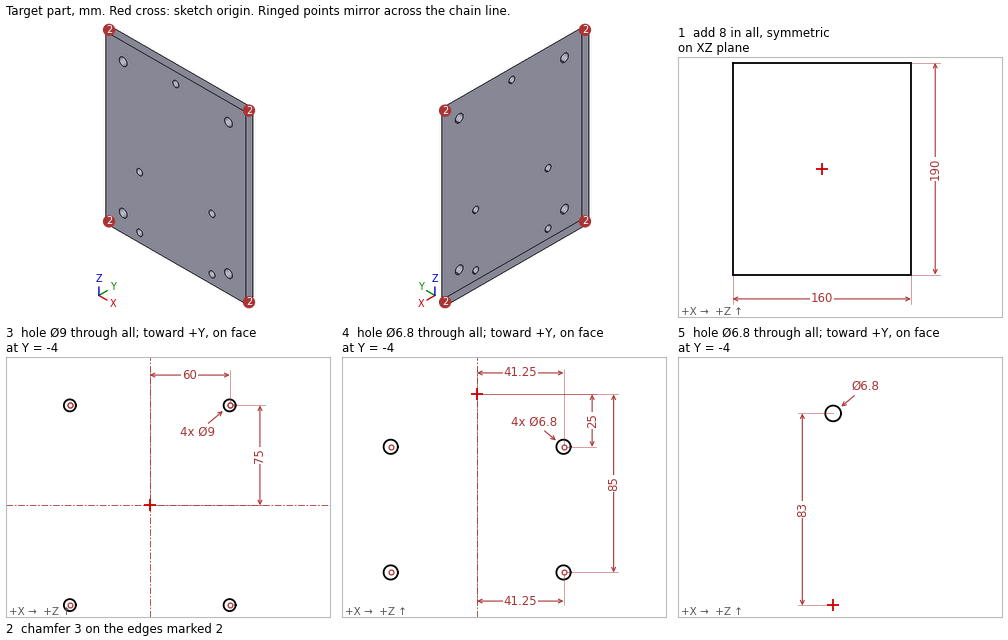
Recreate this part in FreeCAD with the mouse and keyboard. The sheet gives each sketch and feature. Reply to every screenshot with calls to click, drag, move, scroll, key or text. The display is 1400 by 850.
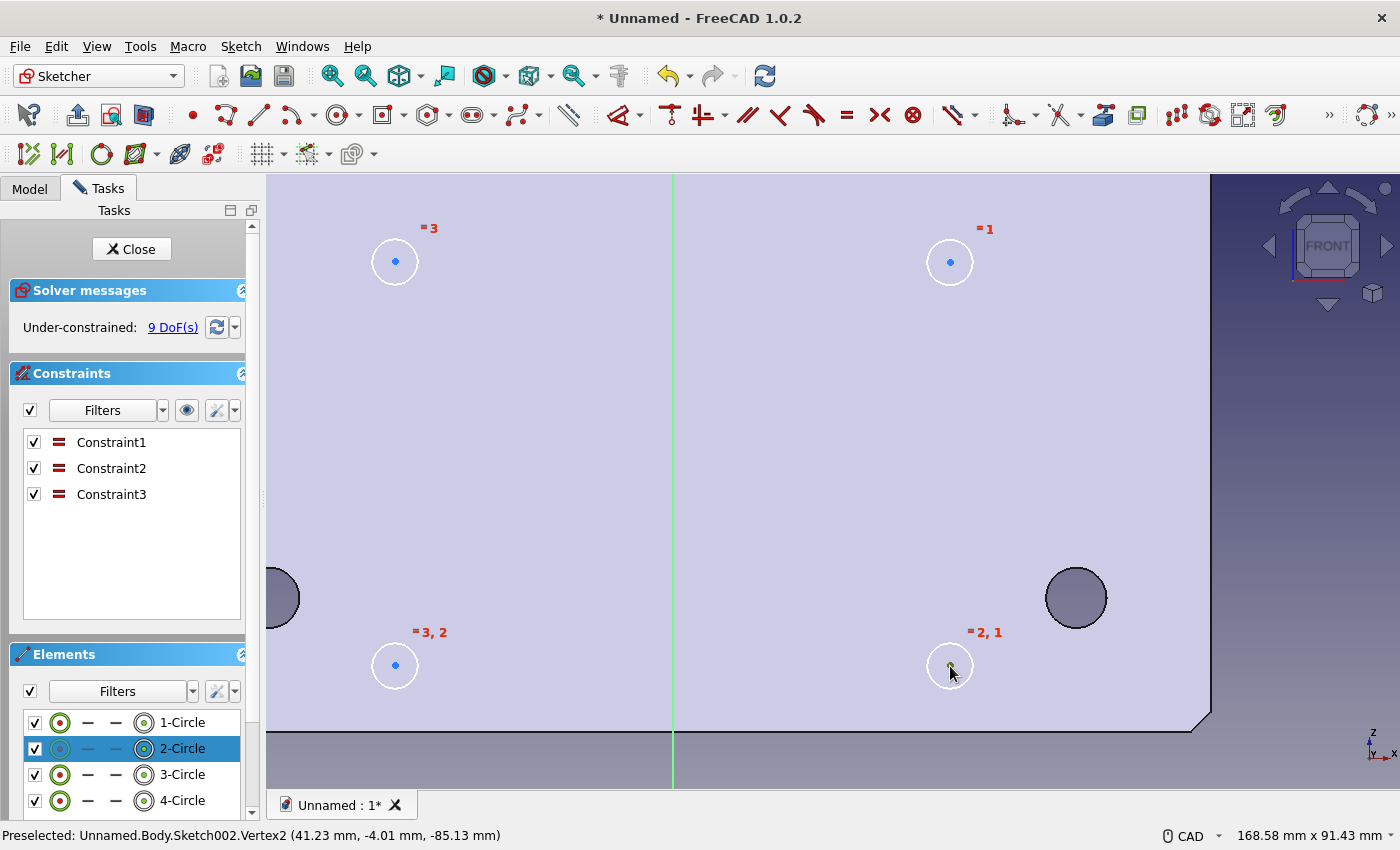
click(395, 666)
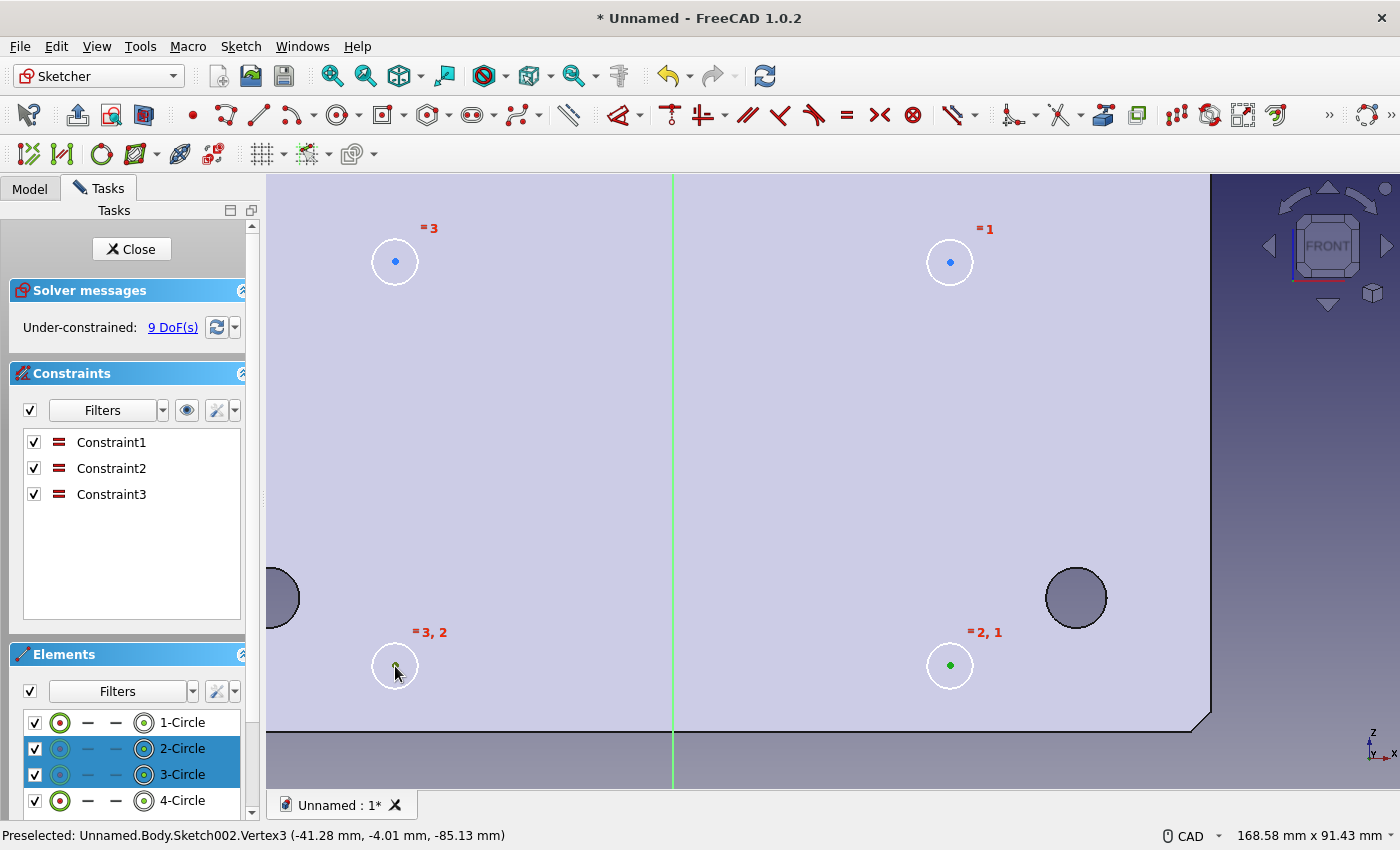
click(673, 721)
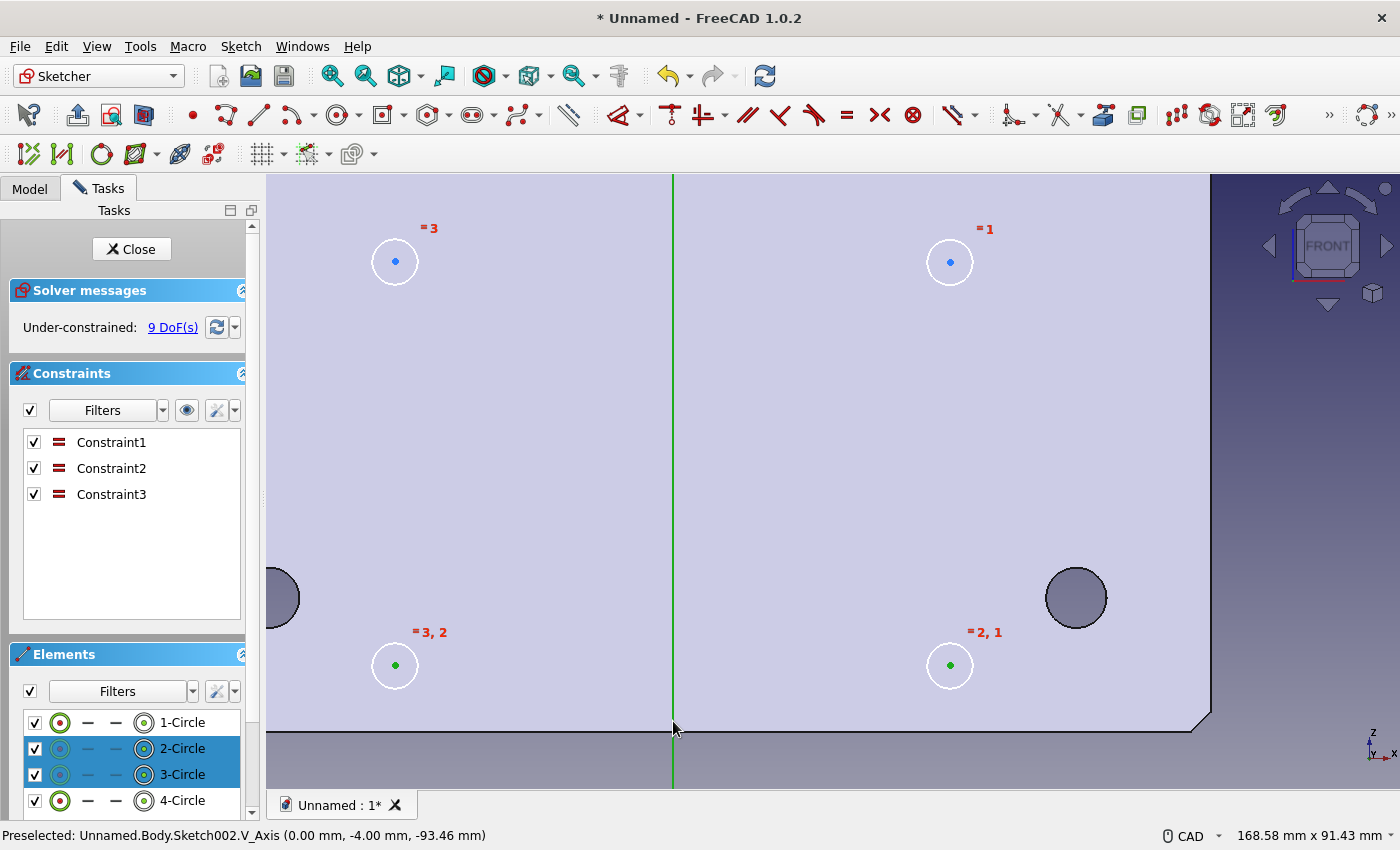
click(880, 116)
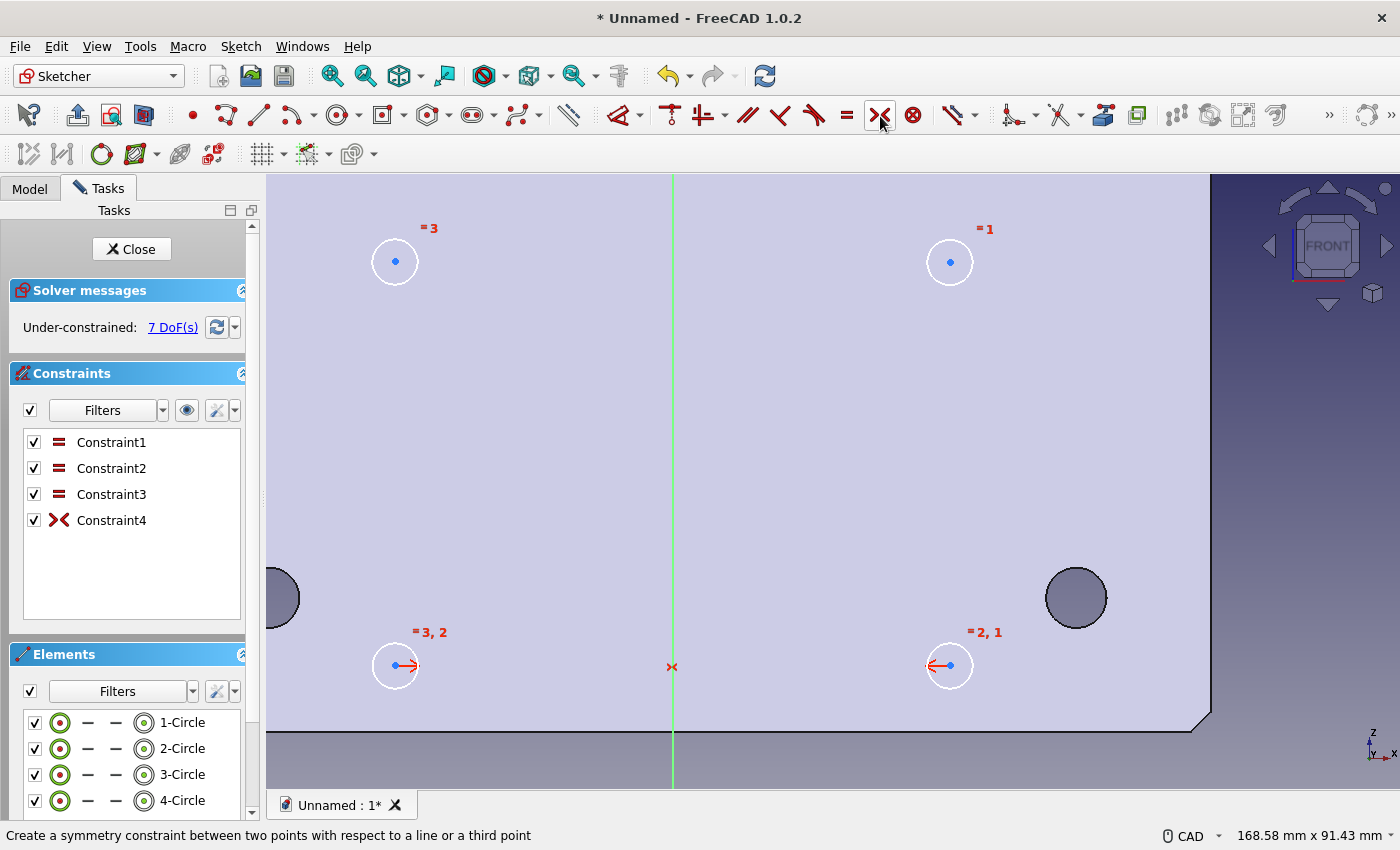
click(950, 262)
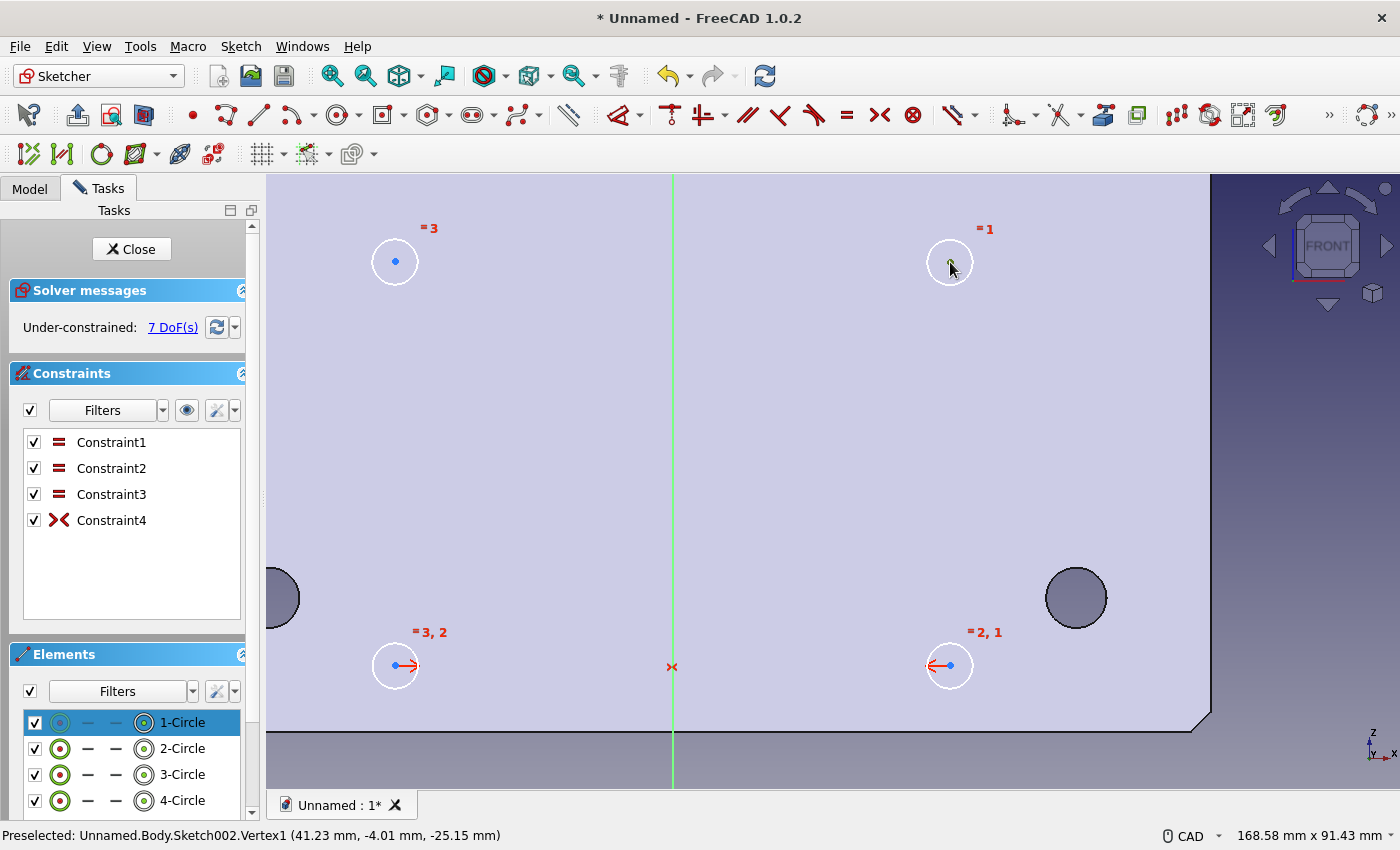
click(395, 262)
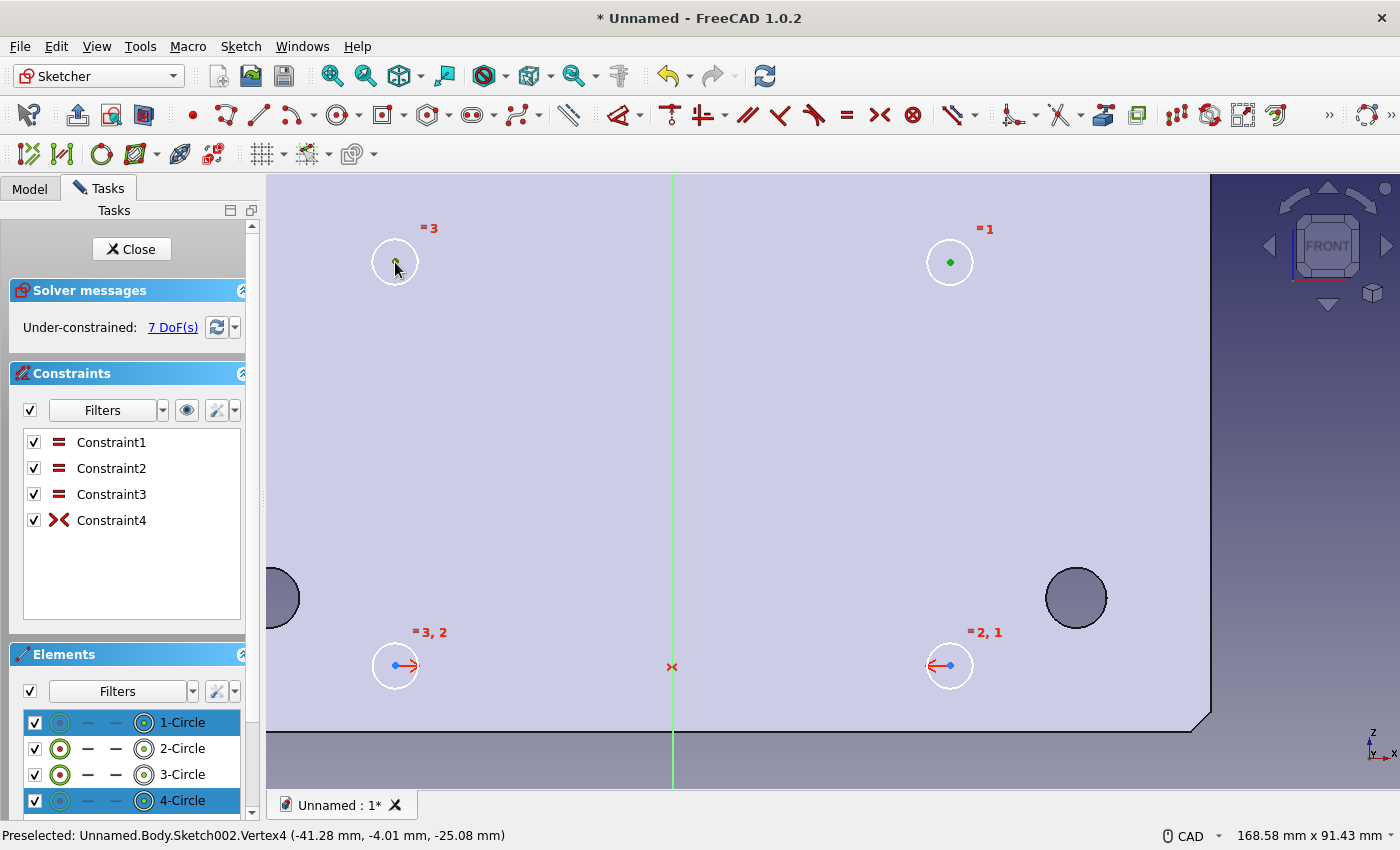
click(673, 721)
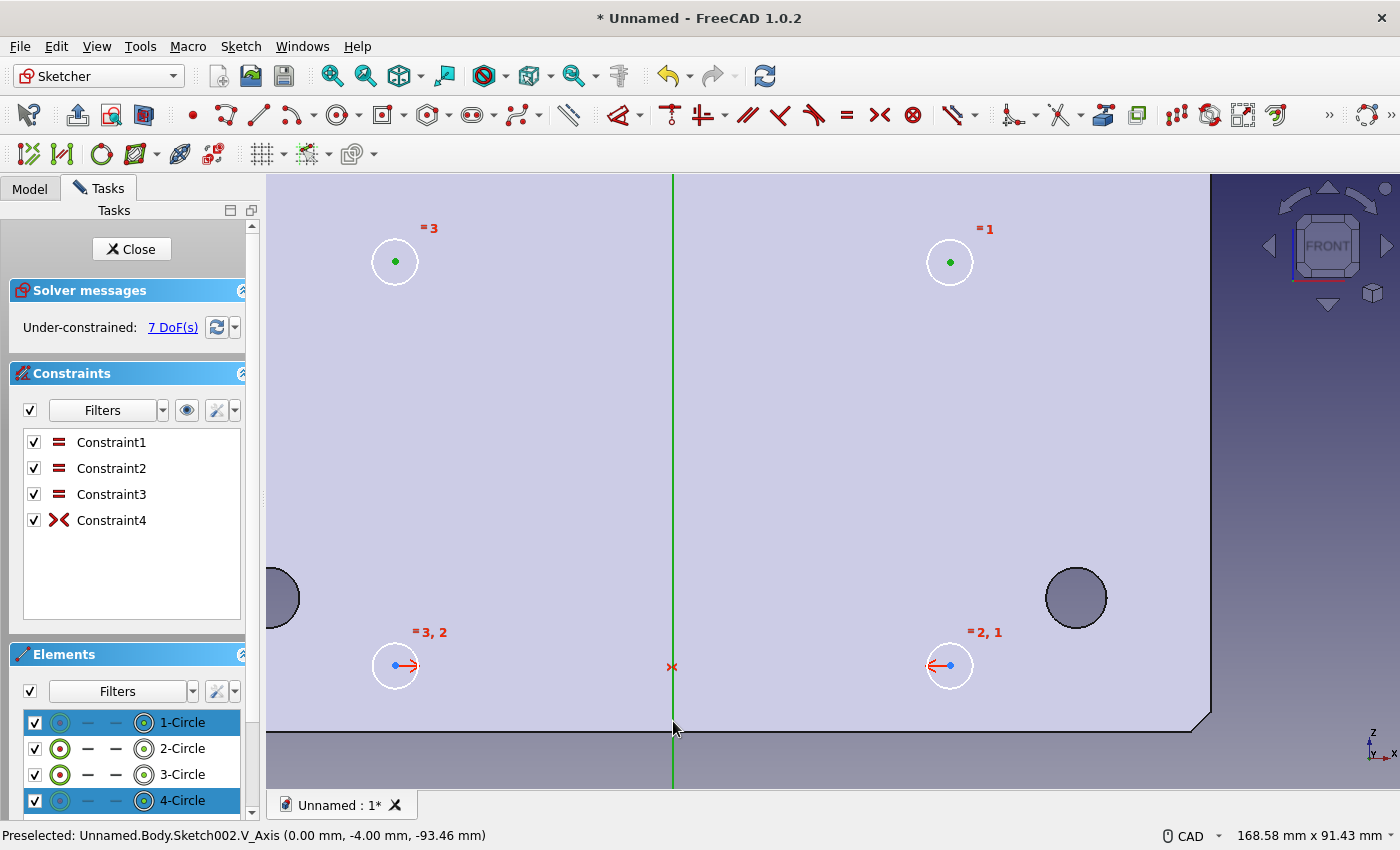
click(880, 116)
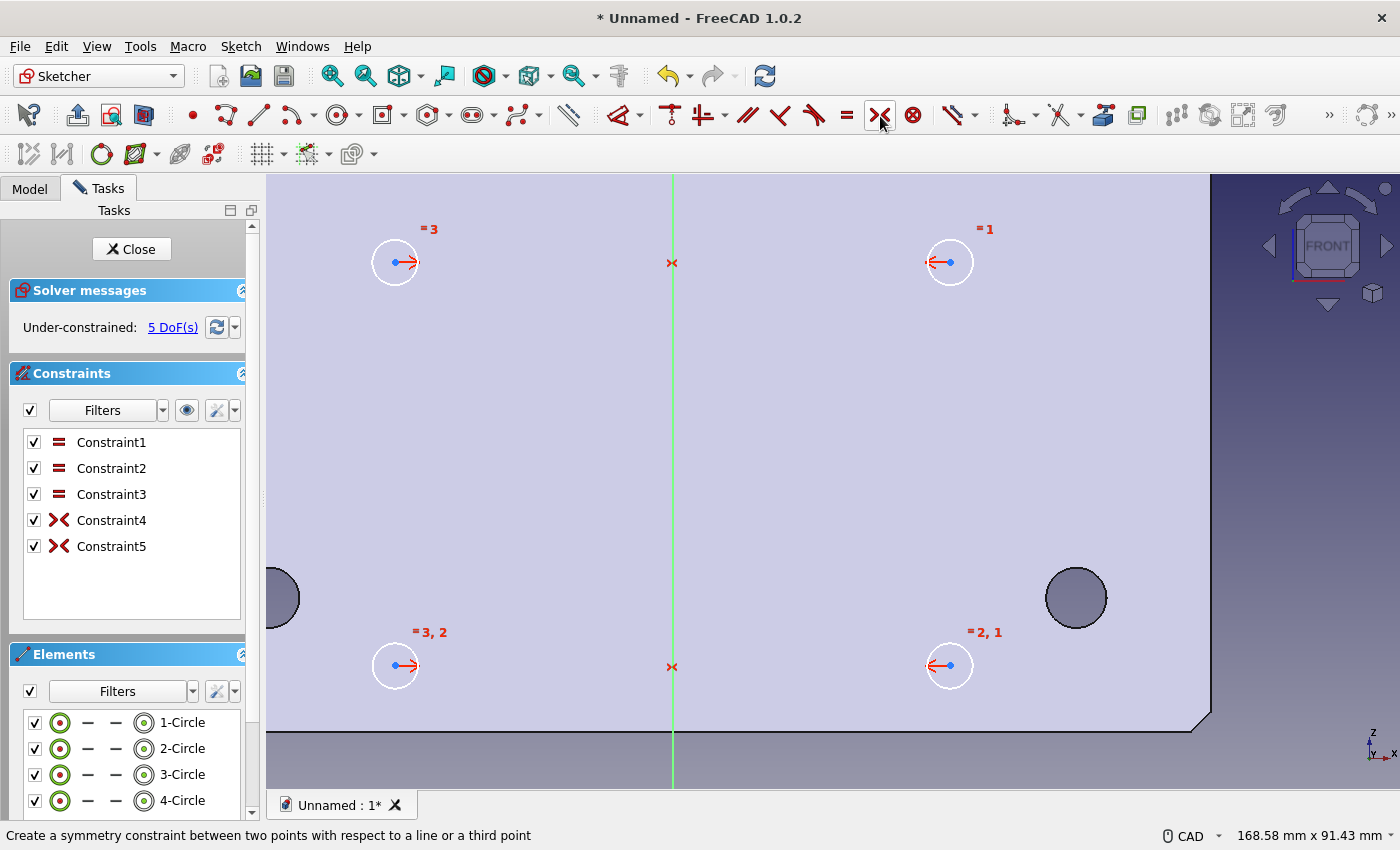
key(d)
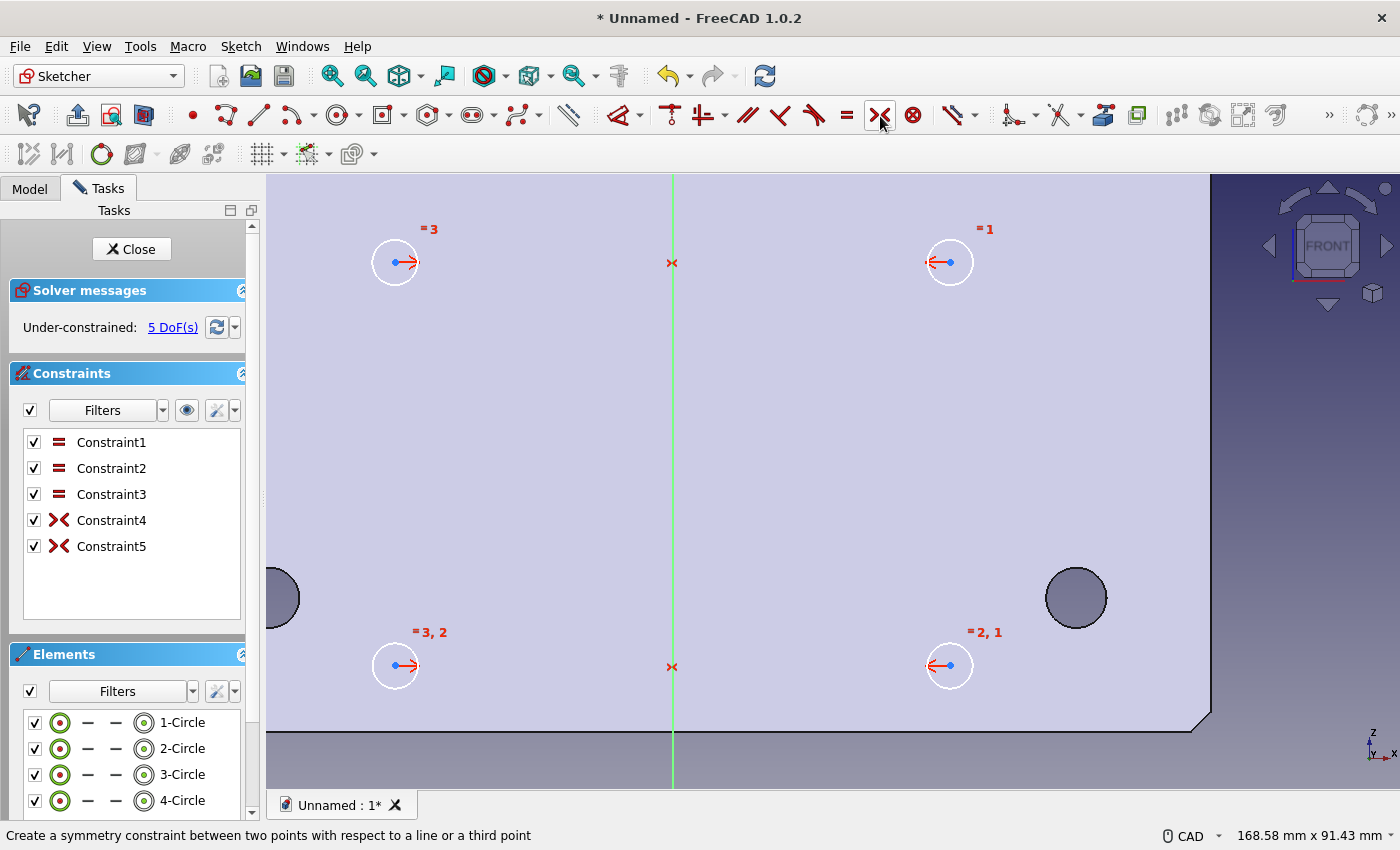
click(966, 246)
click(988, 223)